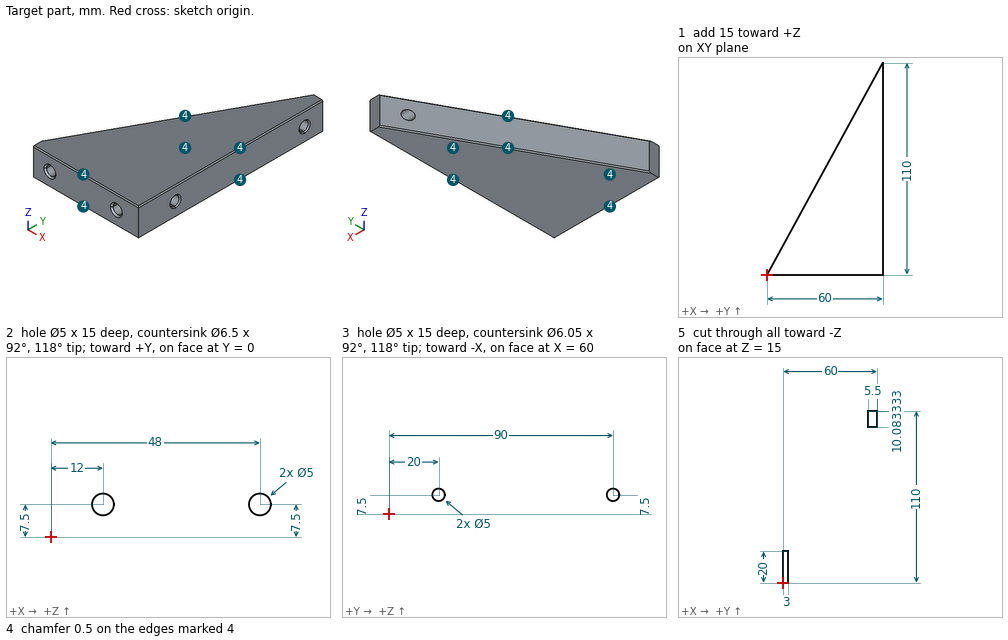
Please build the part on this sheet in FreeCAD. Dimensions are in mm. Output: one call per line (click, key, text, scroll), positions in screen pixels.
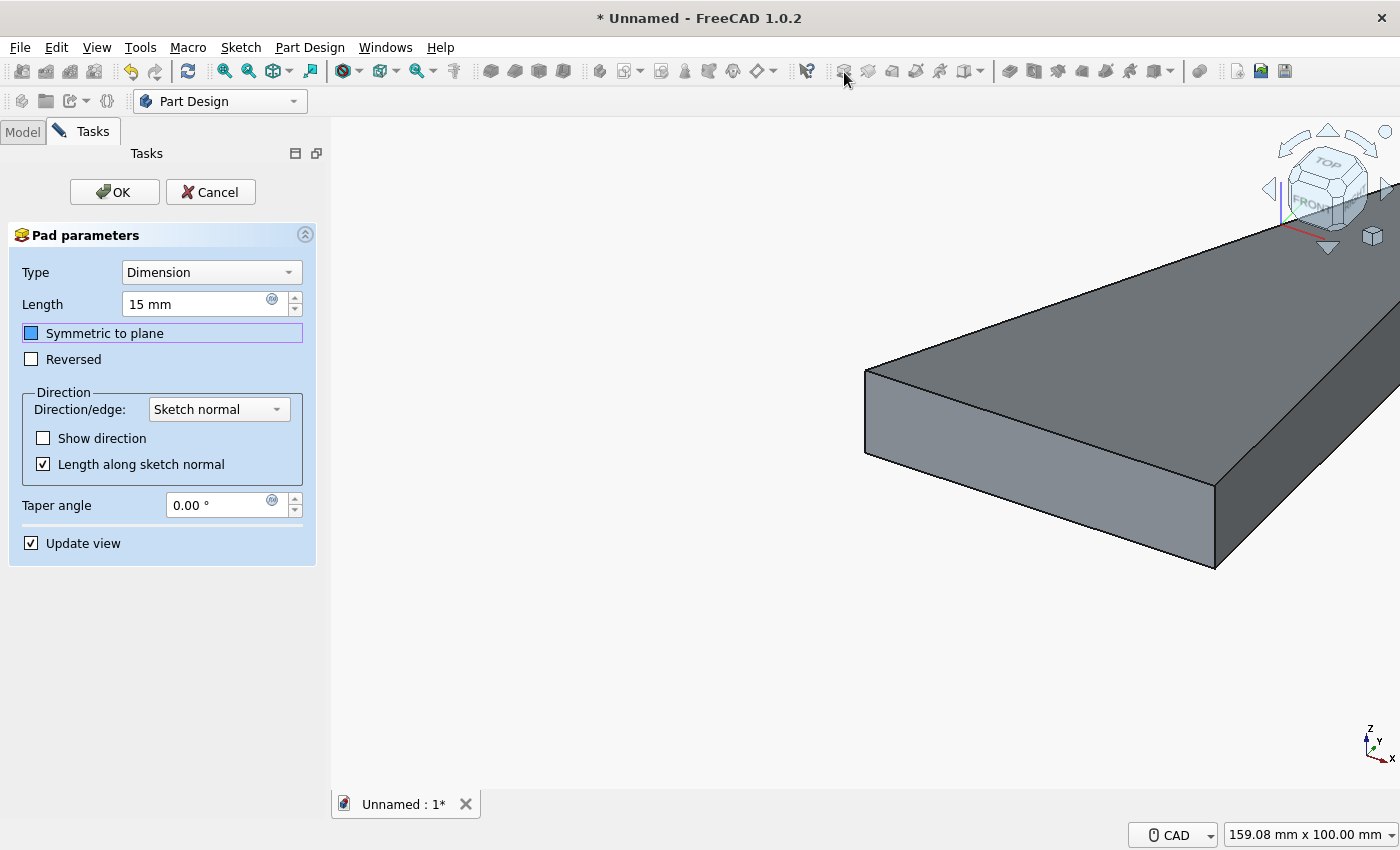
click(115, 192)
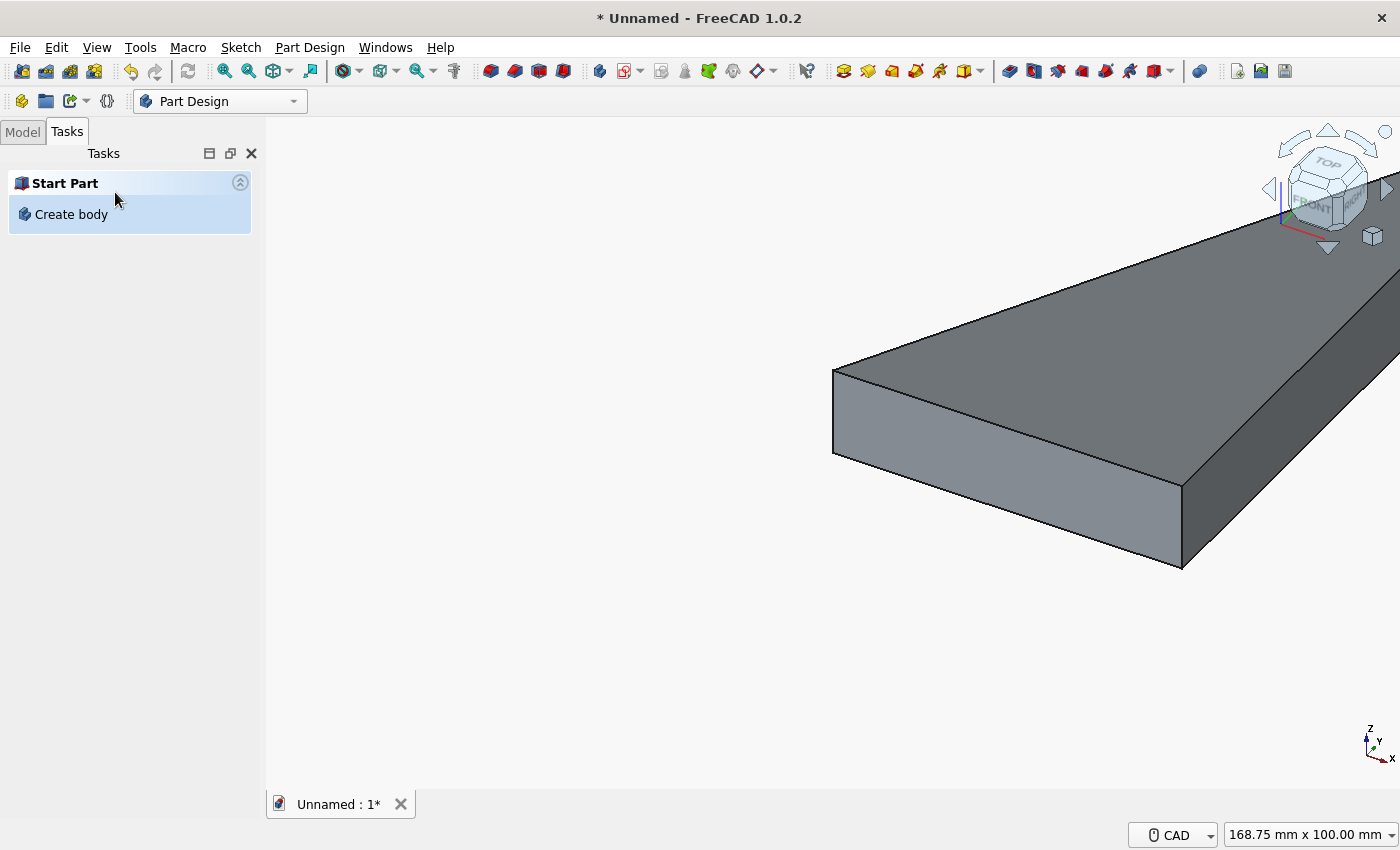
click(226, 72)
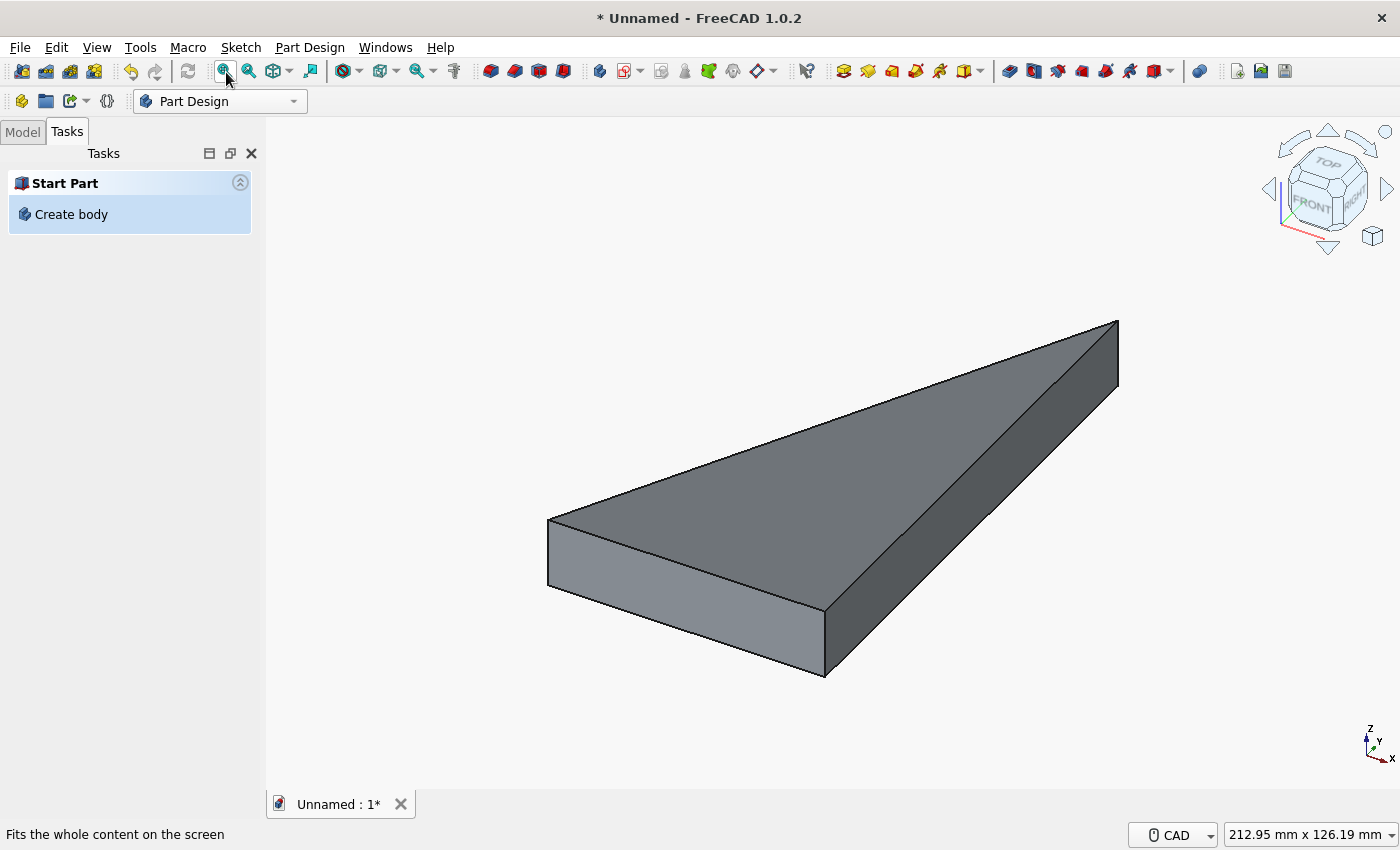
click(766, 624)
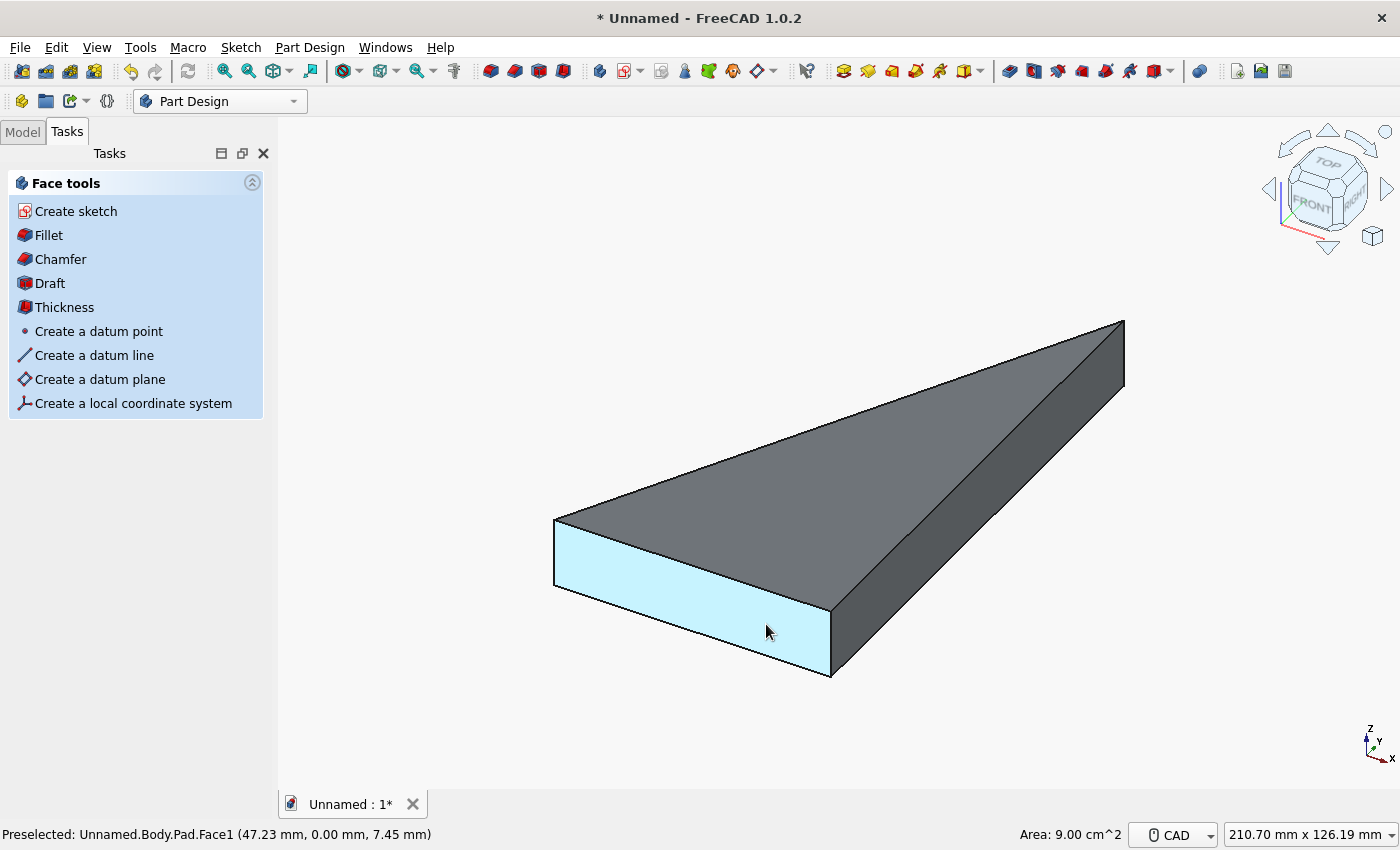
click(624, 72)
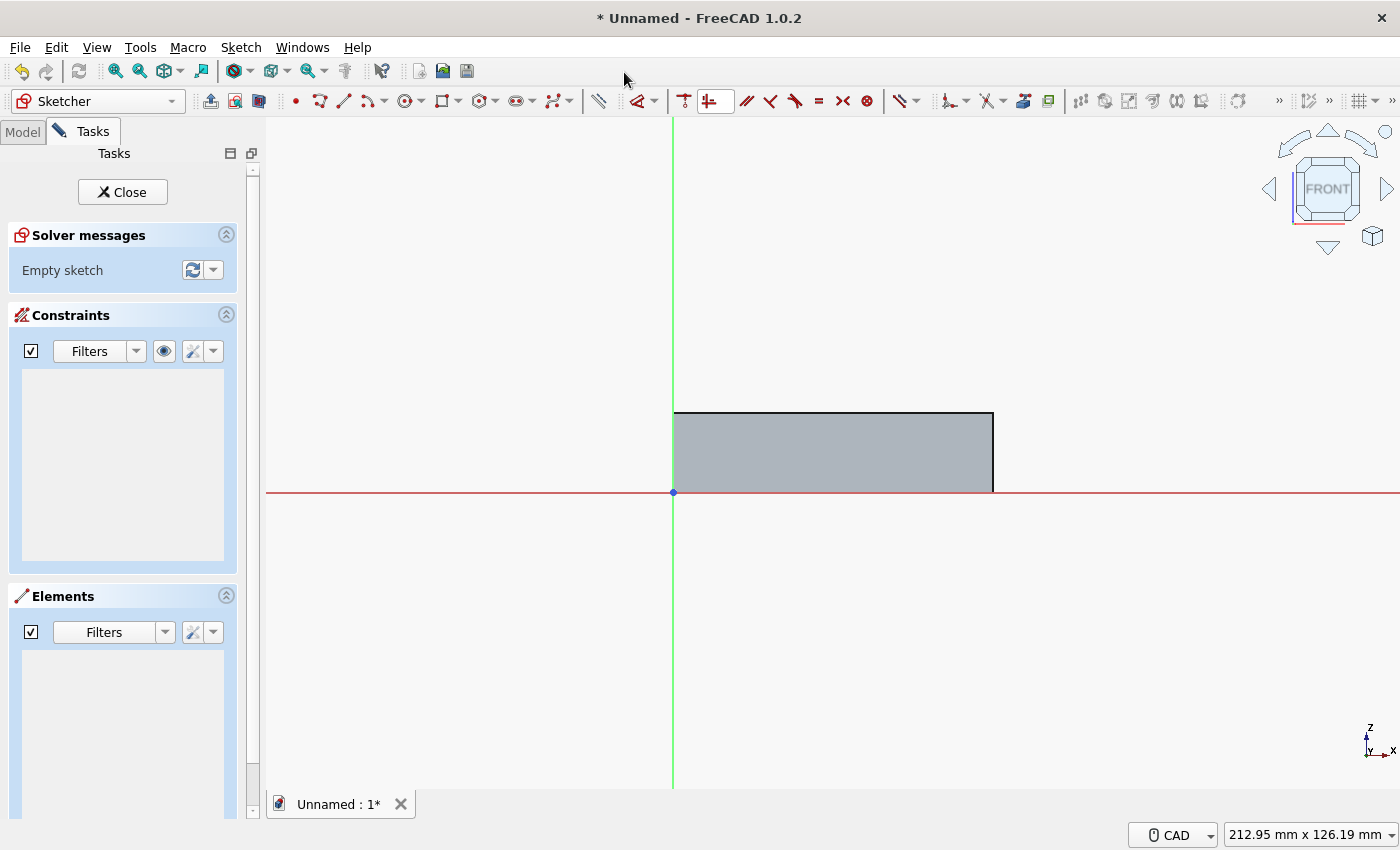
scroll(833, 474, up, 5)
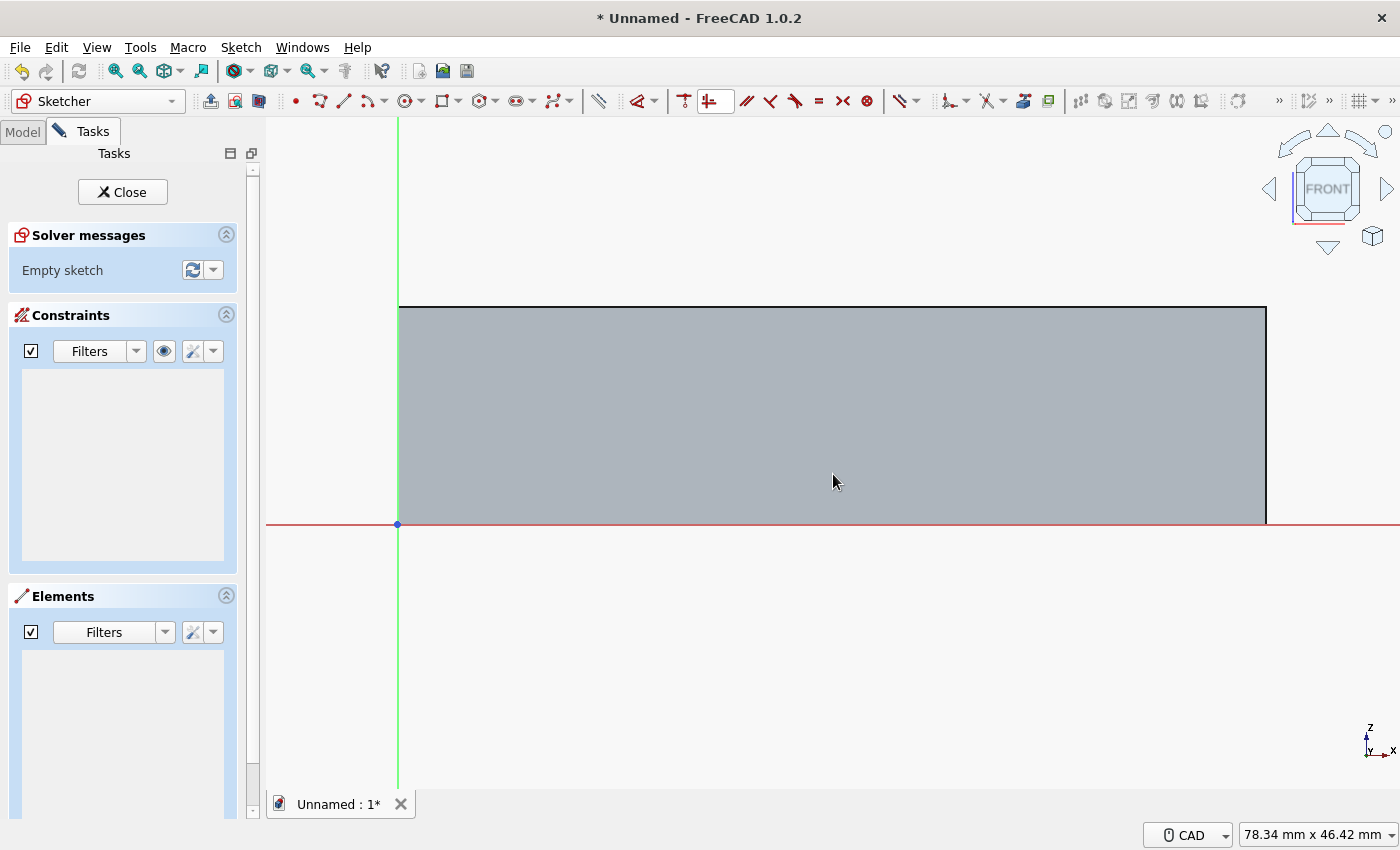
key(g)
key(c)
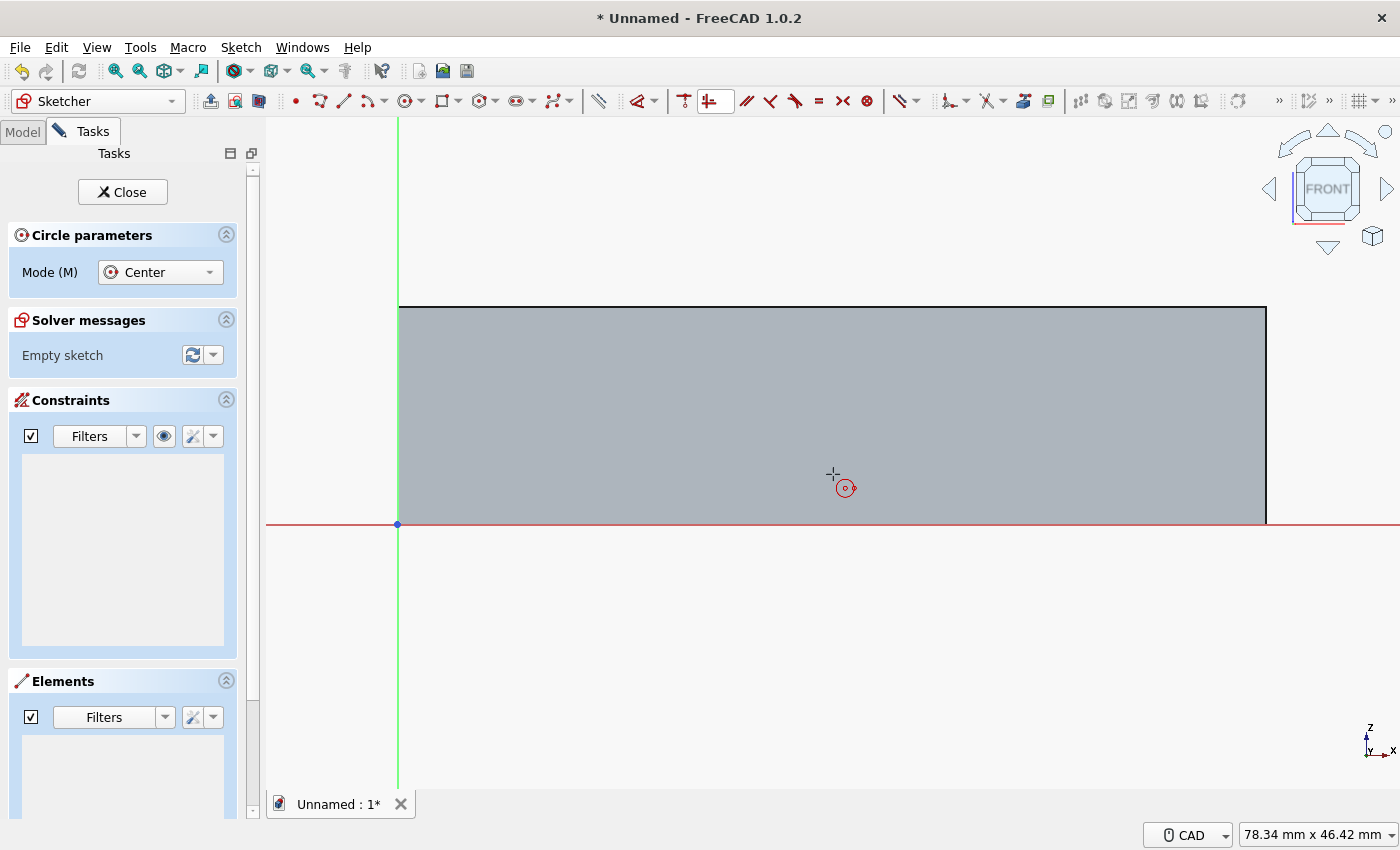
click(1093, 416)
click(1118, 390)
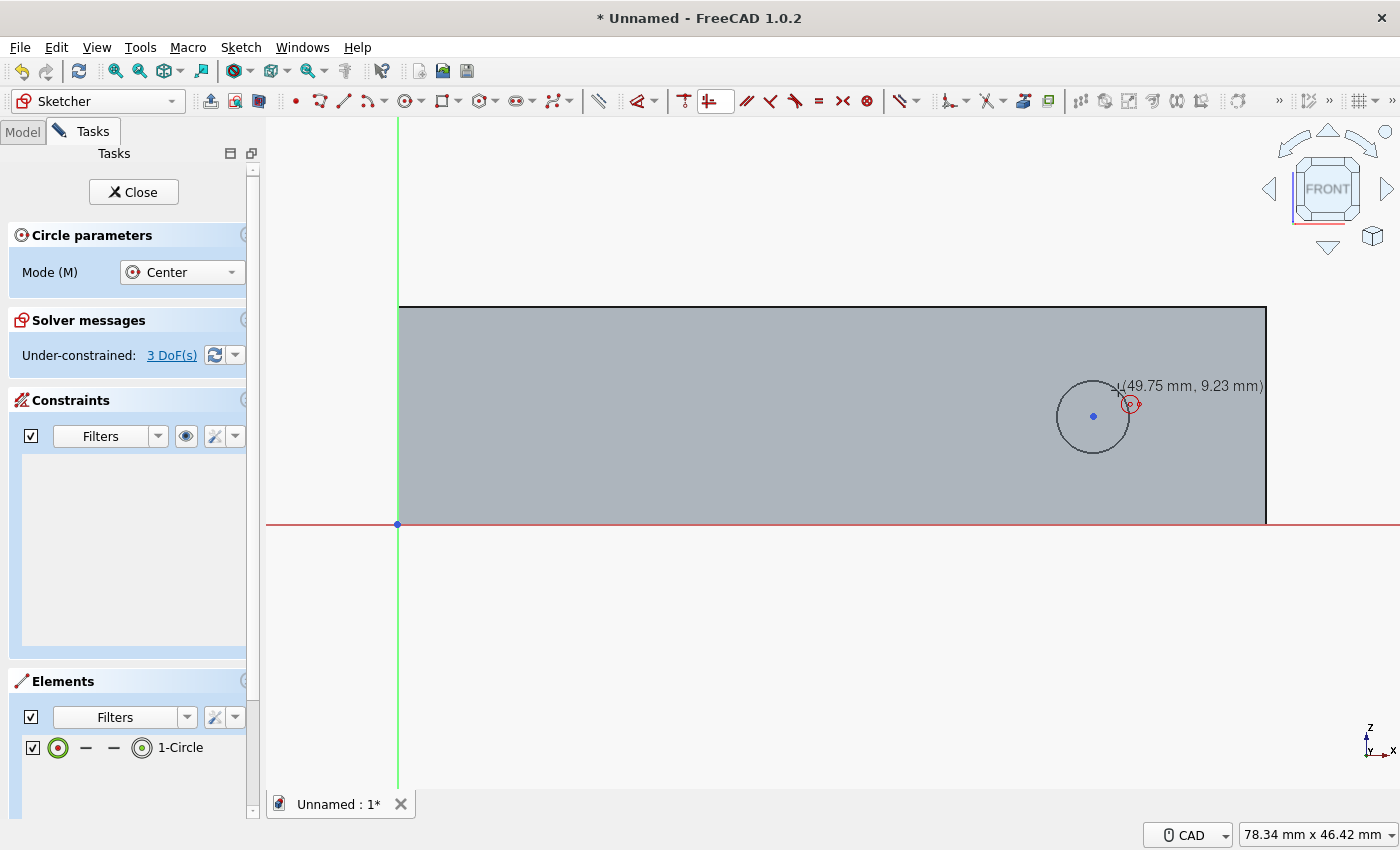
click(572, 416)
click(597, 390)
key(Escape)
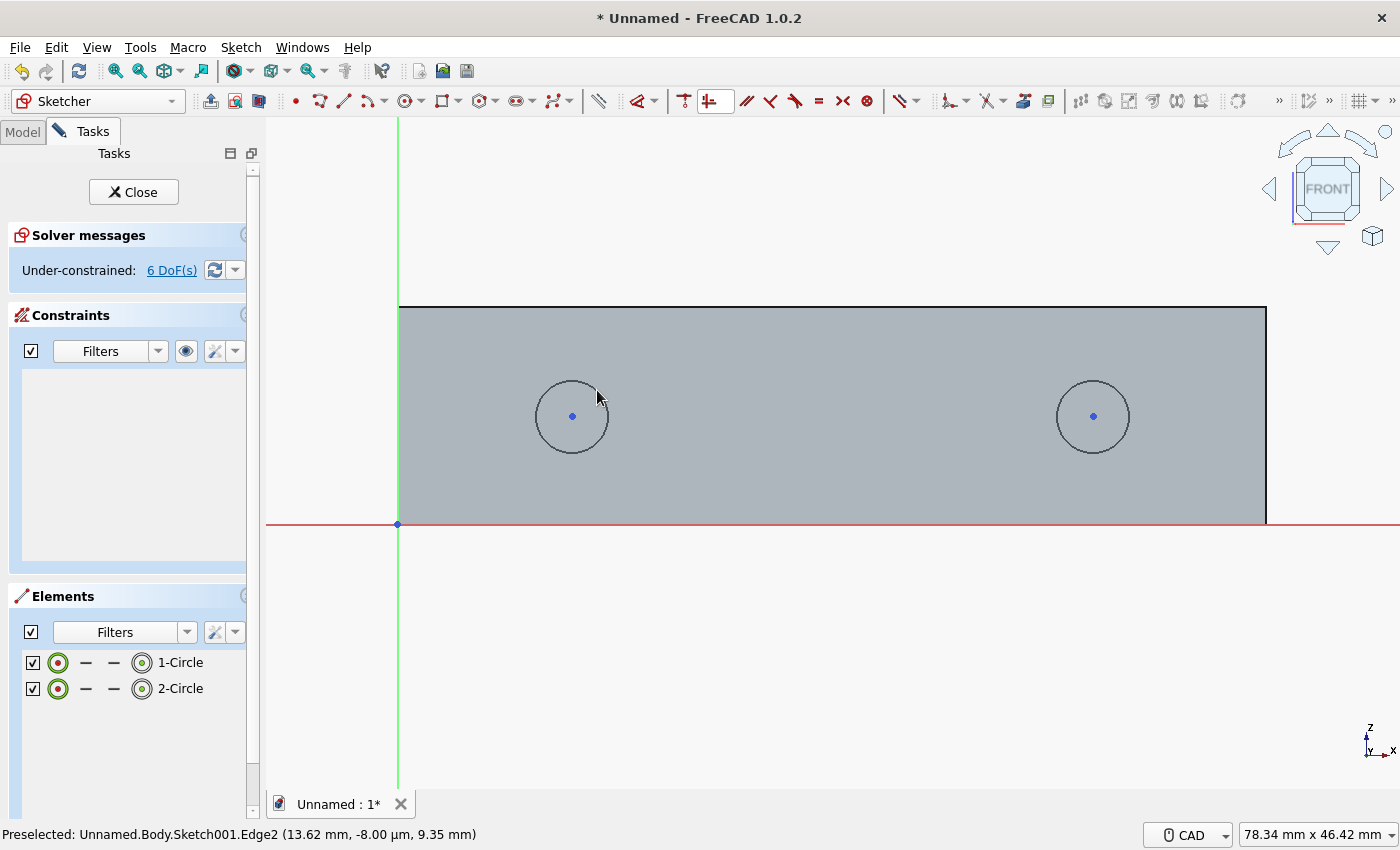
click(1118, 391)